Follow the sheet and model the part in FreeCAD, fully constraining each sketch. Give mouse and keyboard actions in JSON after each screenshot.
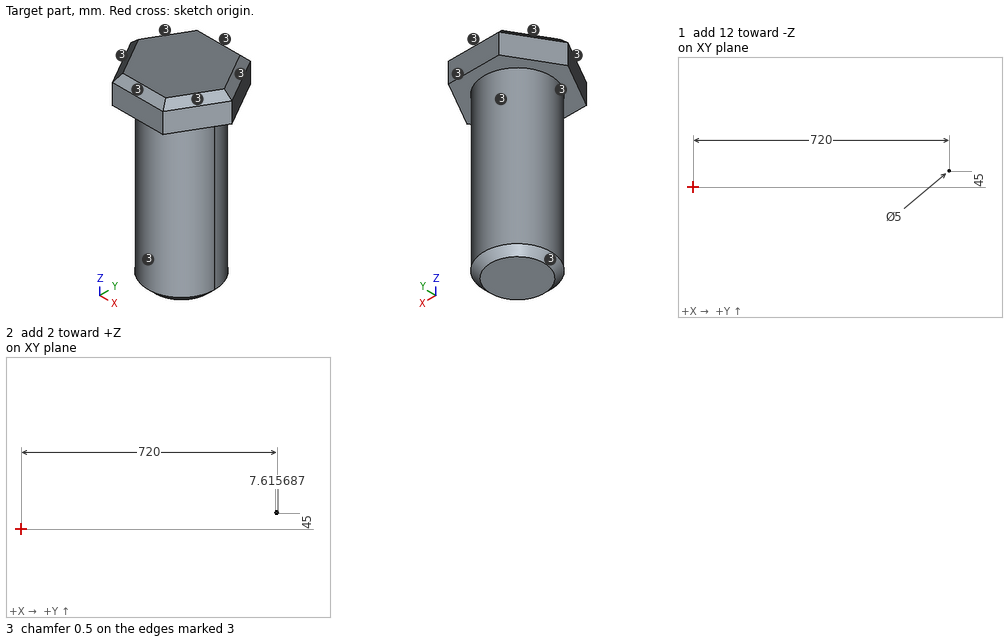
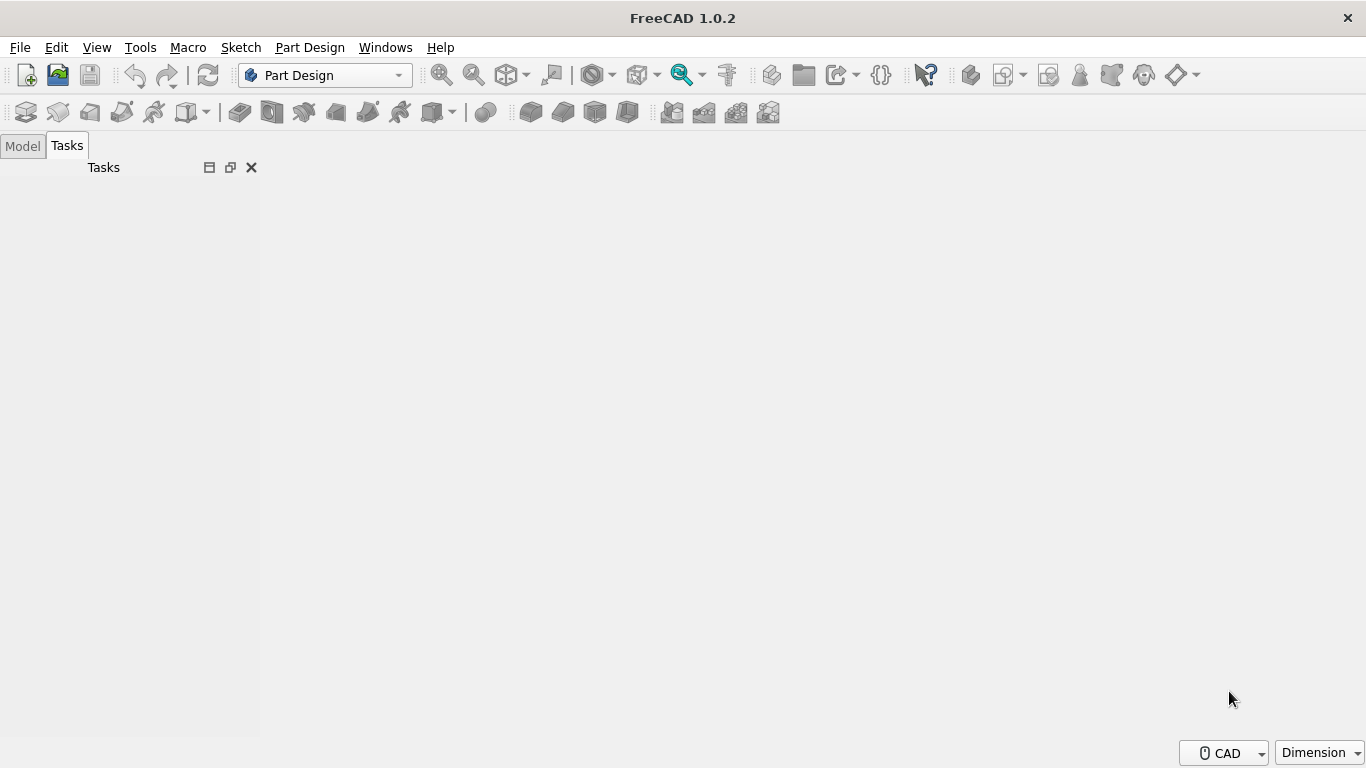
{"action": "left_click", "coordinate": [26, 76]}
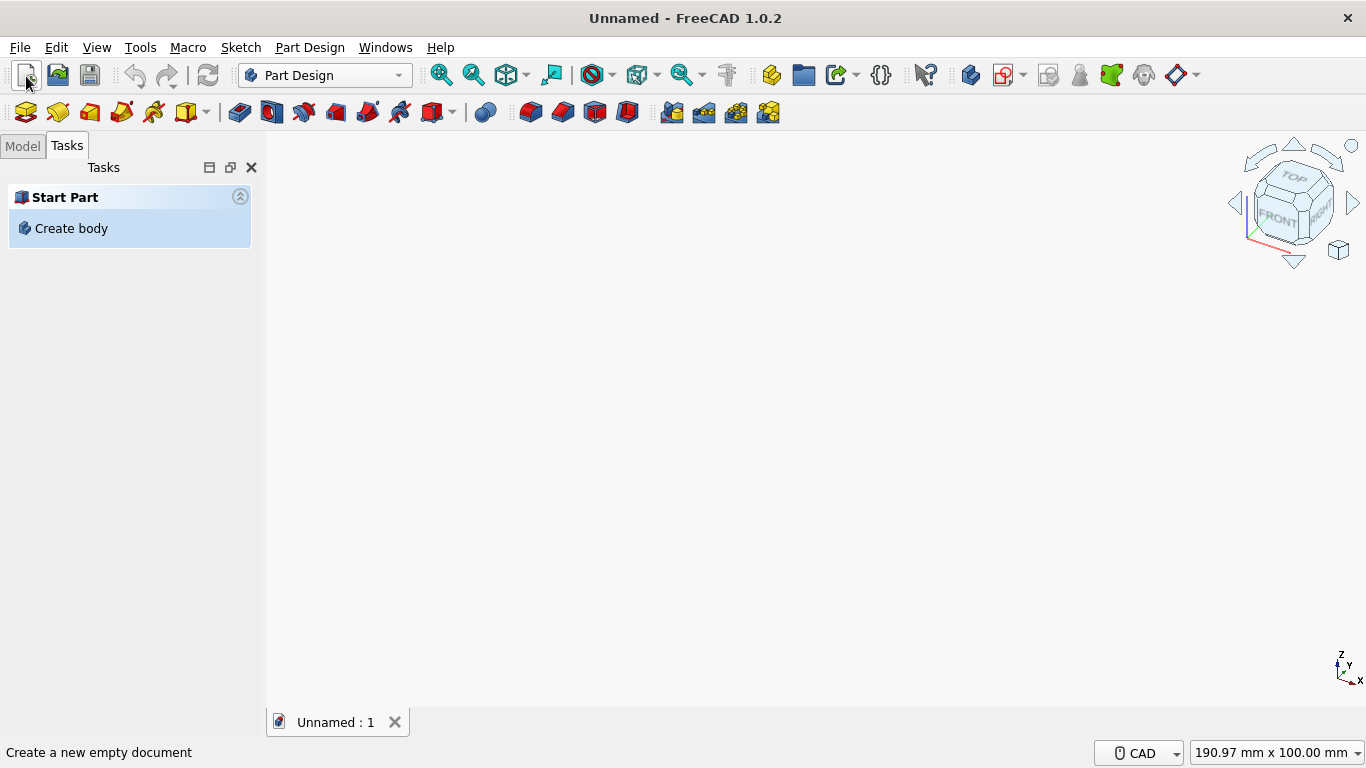
{"action": "left_click", "coordinate": [1004, 76]}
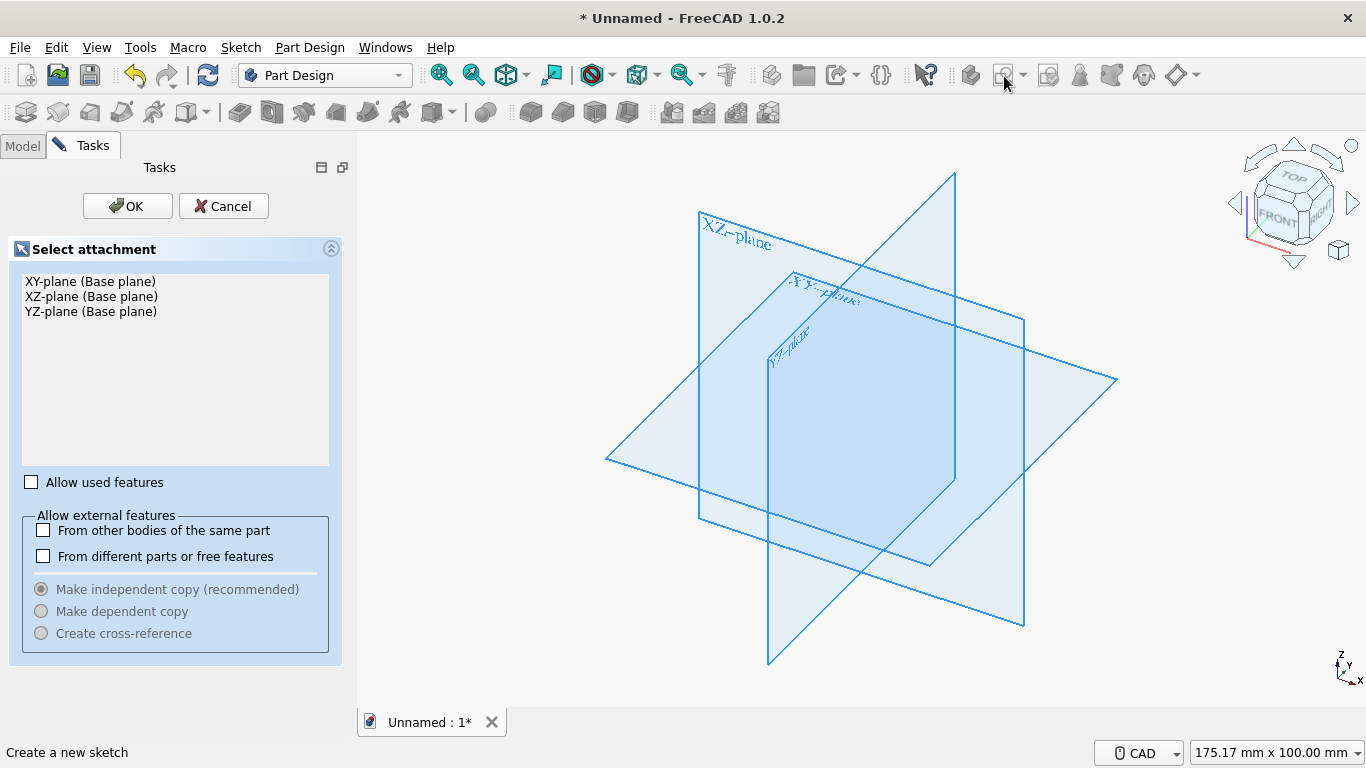
{"action": "left_click", "coordinate": [82, 282]}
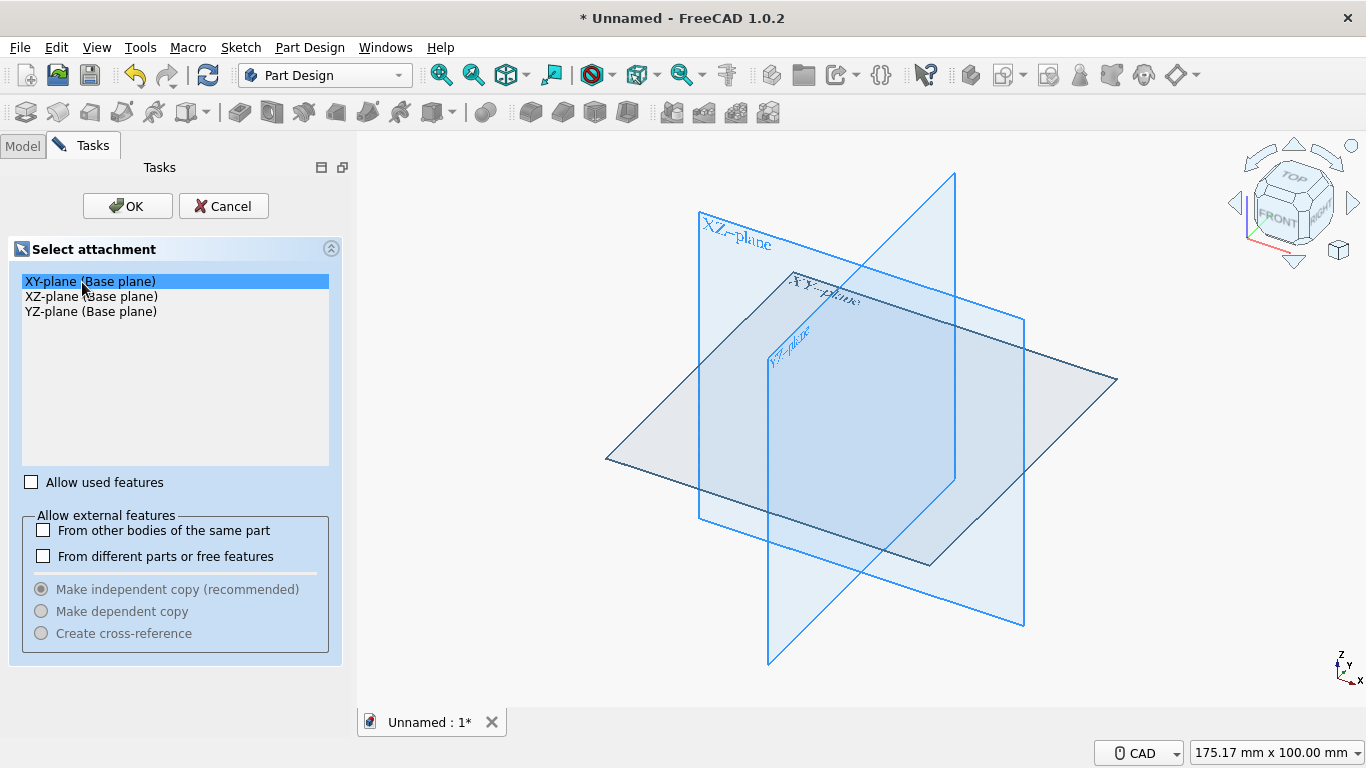
{"action": "left_click", "coordinate": [128, 206]}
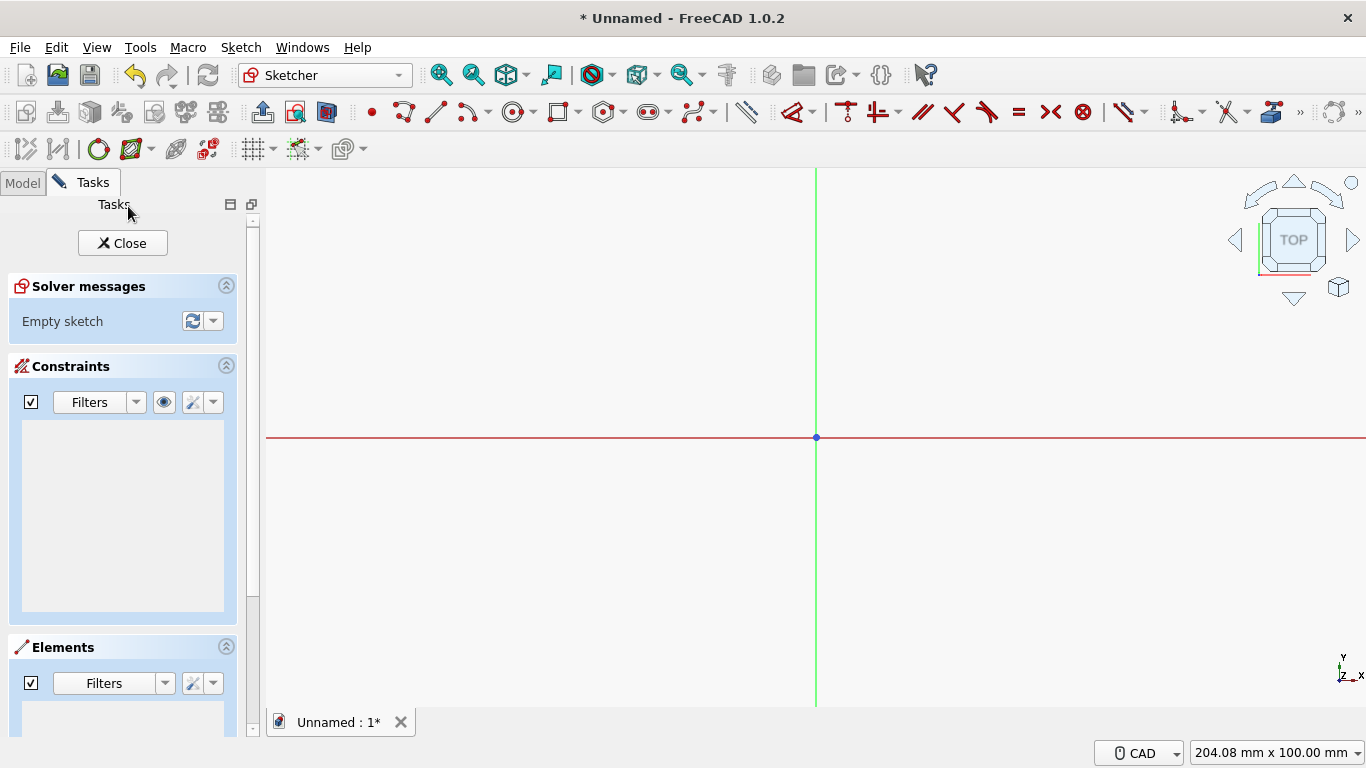
{"action": "scroll", "coordinate": [748, 438], "scroll_direction": "down", "scroll_amount": 5}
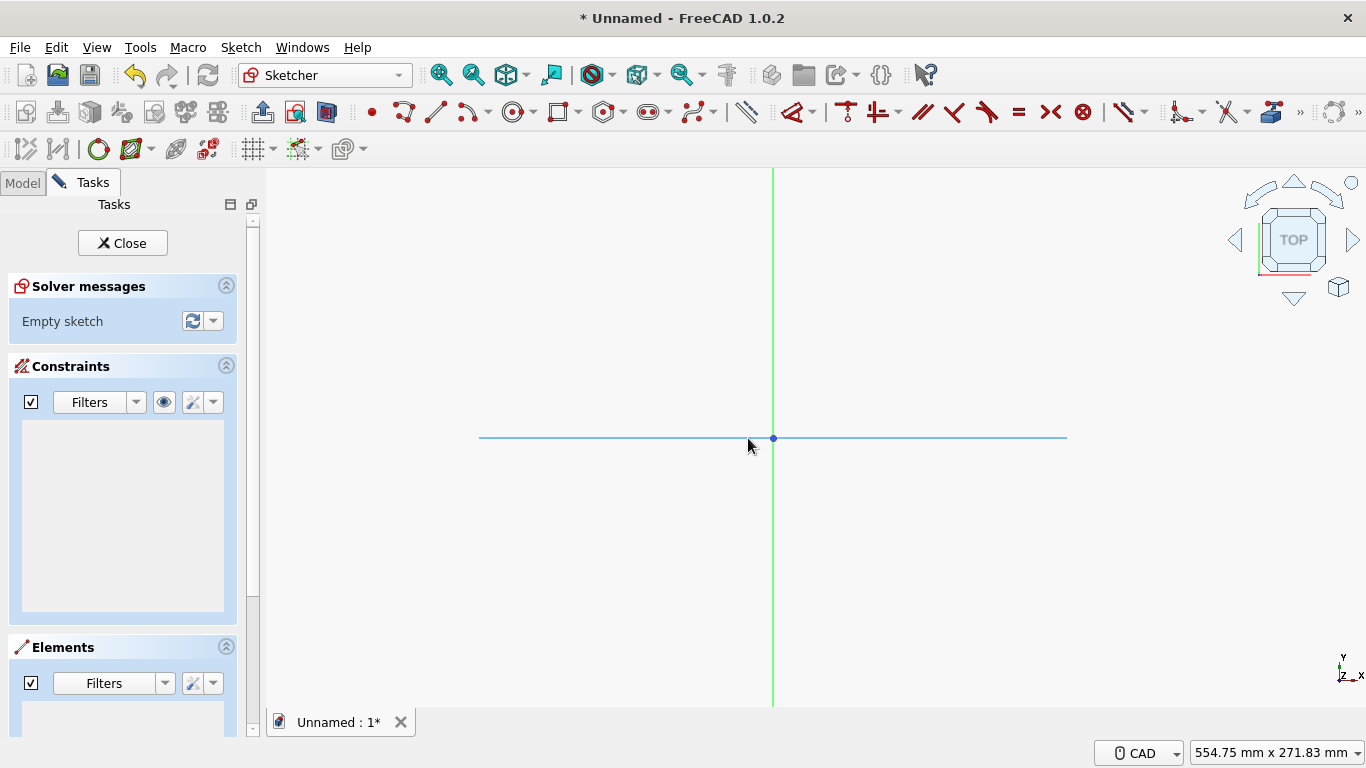
{"action": "scroll", "coordinate": [748, 438], "scroll_direction": "down", "scroll_amount": 5}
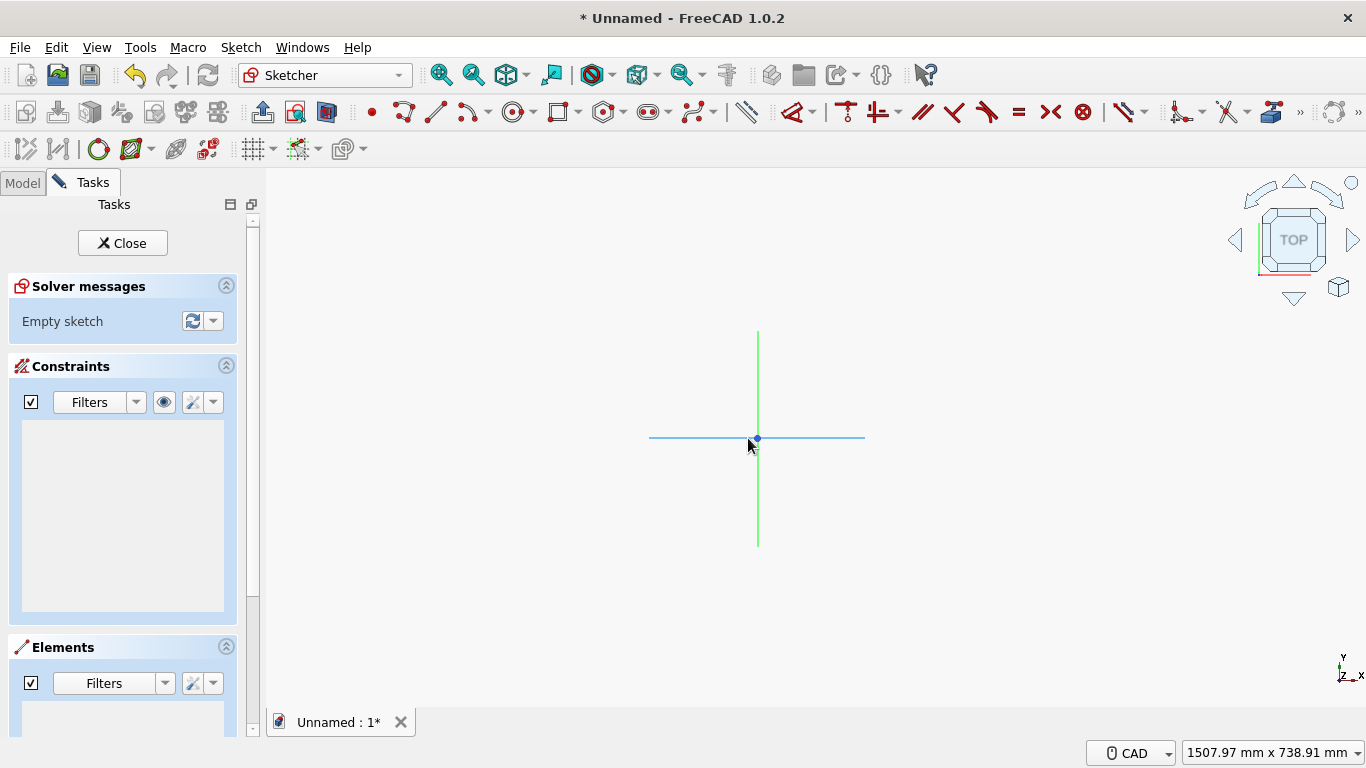
{"action": "scroll", "coordinate": [748, 438], "scroll_direction": "down", "scroll_amount": 5}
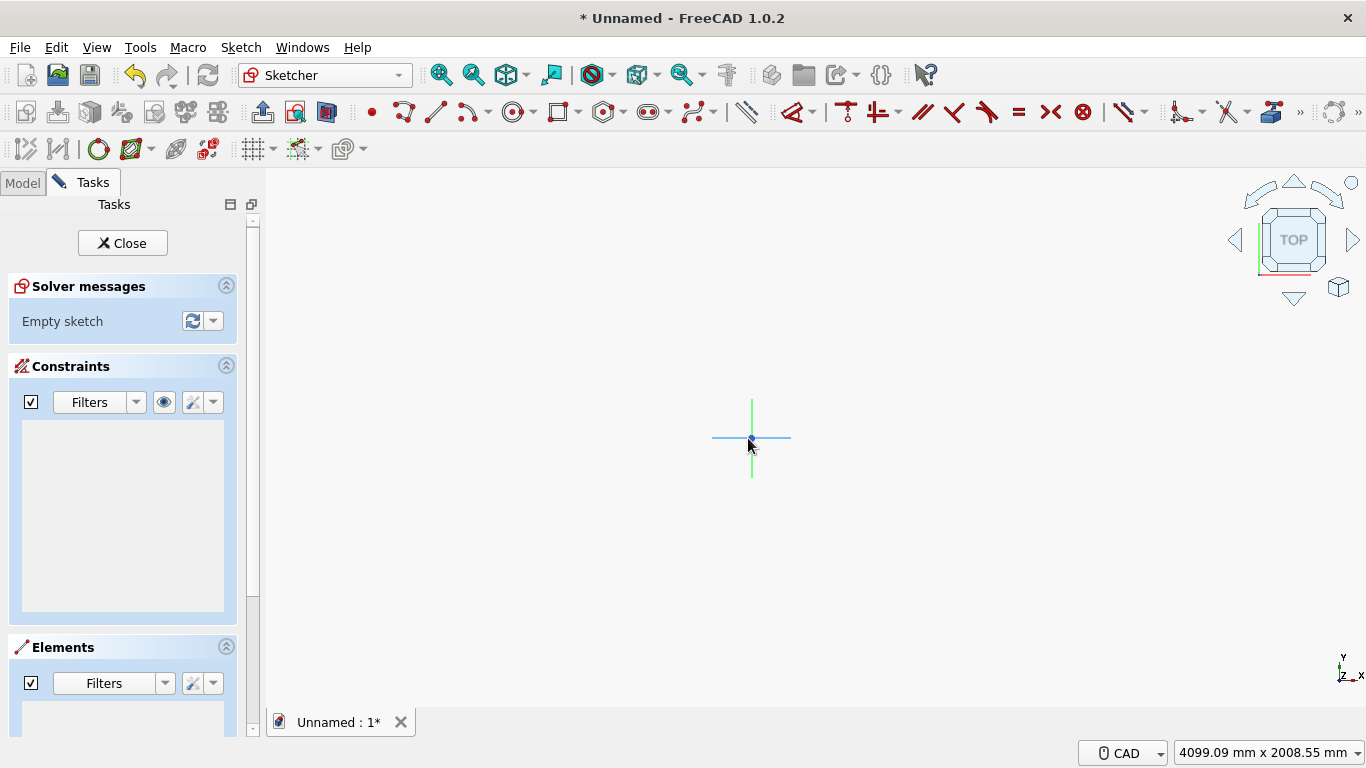
{"action": "scroll", "coordinate": [955, 426], "scroll_direction": "up", "scroll_amount": 15}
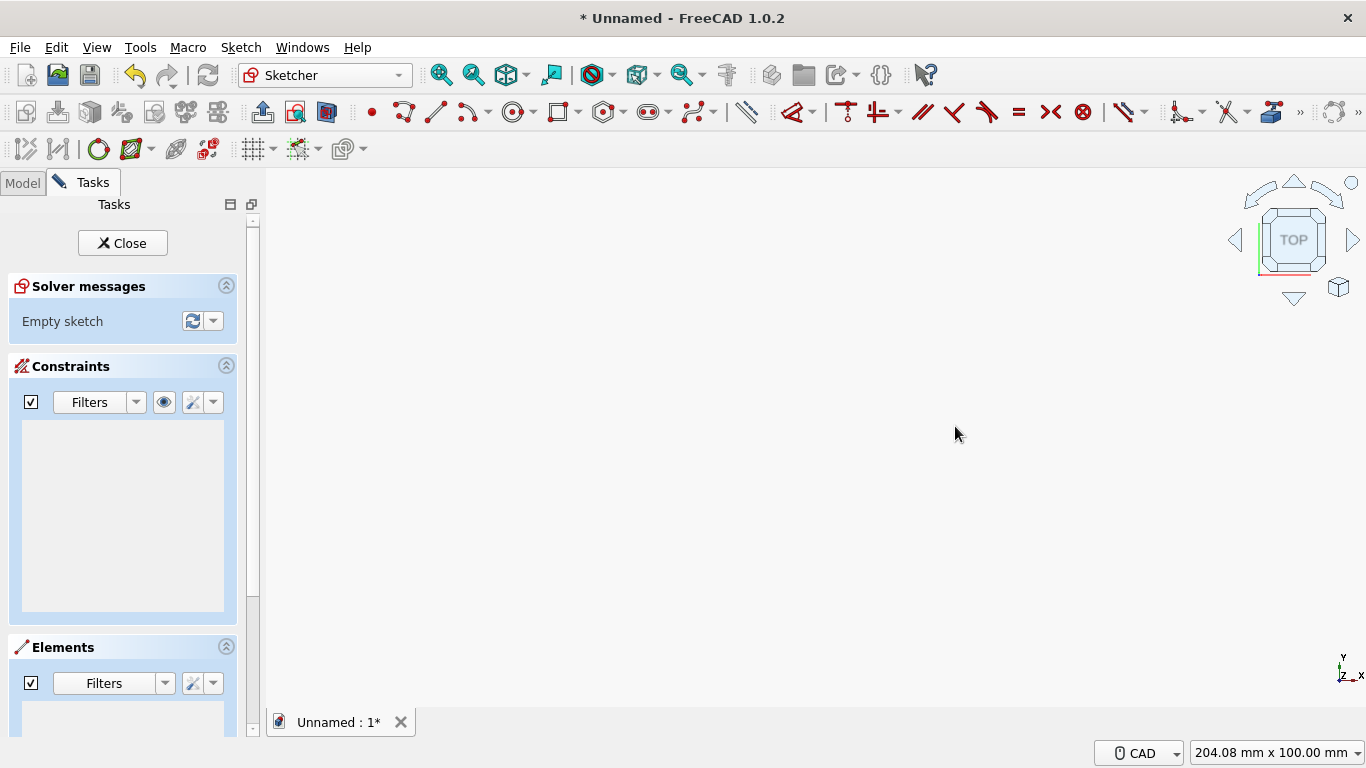
{"action": "scroll", "coordinate": [742, 423], "scroll_direction": "up", "scroll_amount": 13}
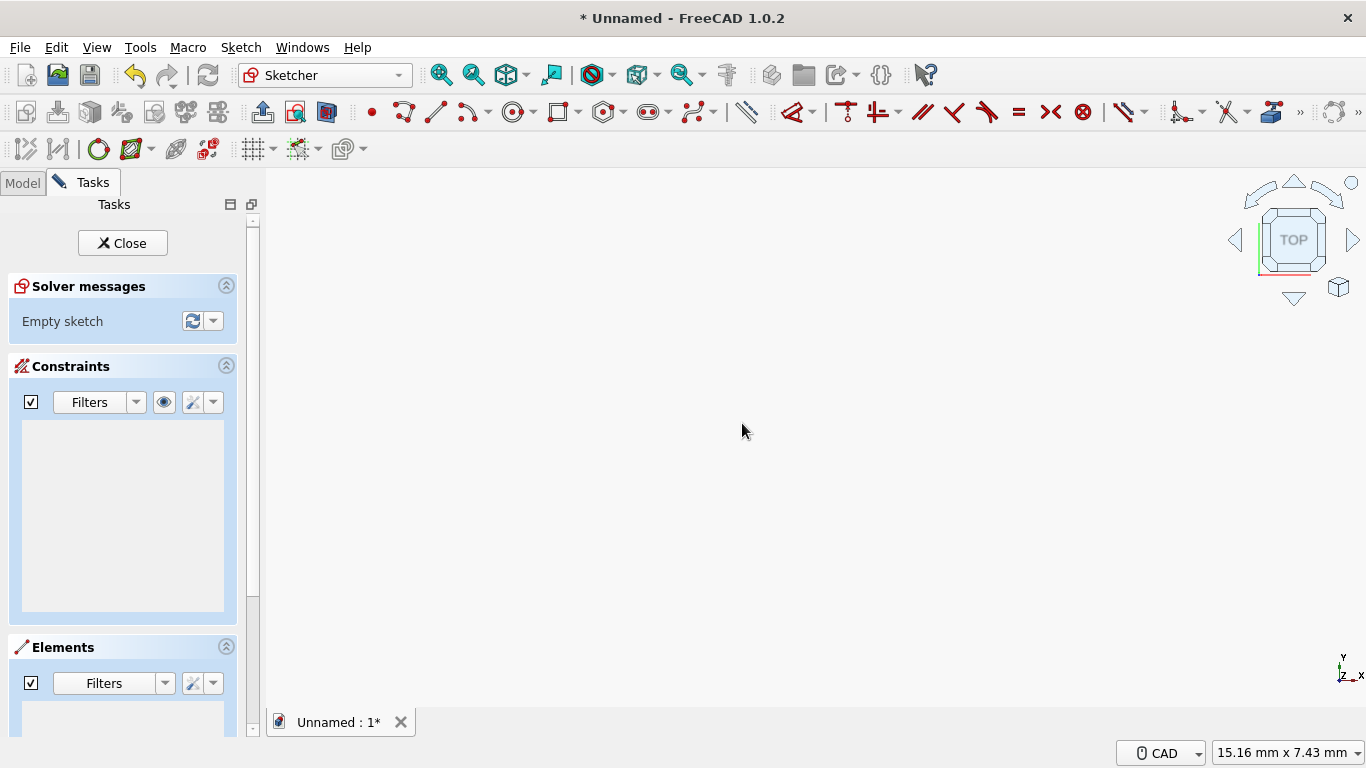
{"action": "left_click", "coordinate": [514, 112]}